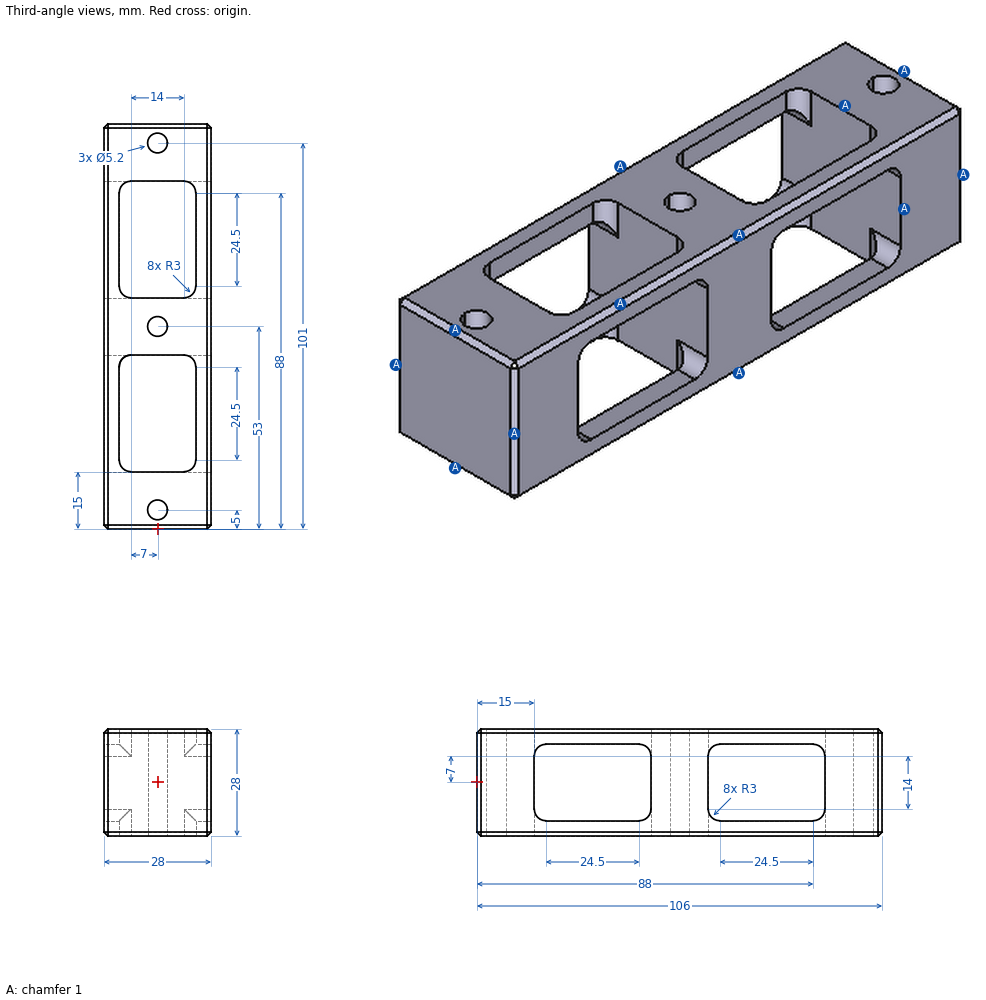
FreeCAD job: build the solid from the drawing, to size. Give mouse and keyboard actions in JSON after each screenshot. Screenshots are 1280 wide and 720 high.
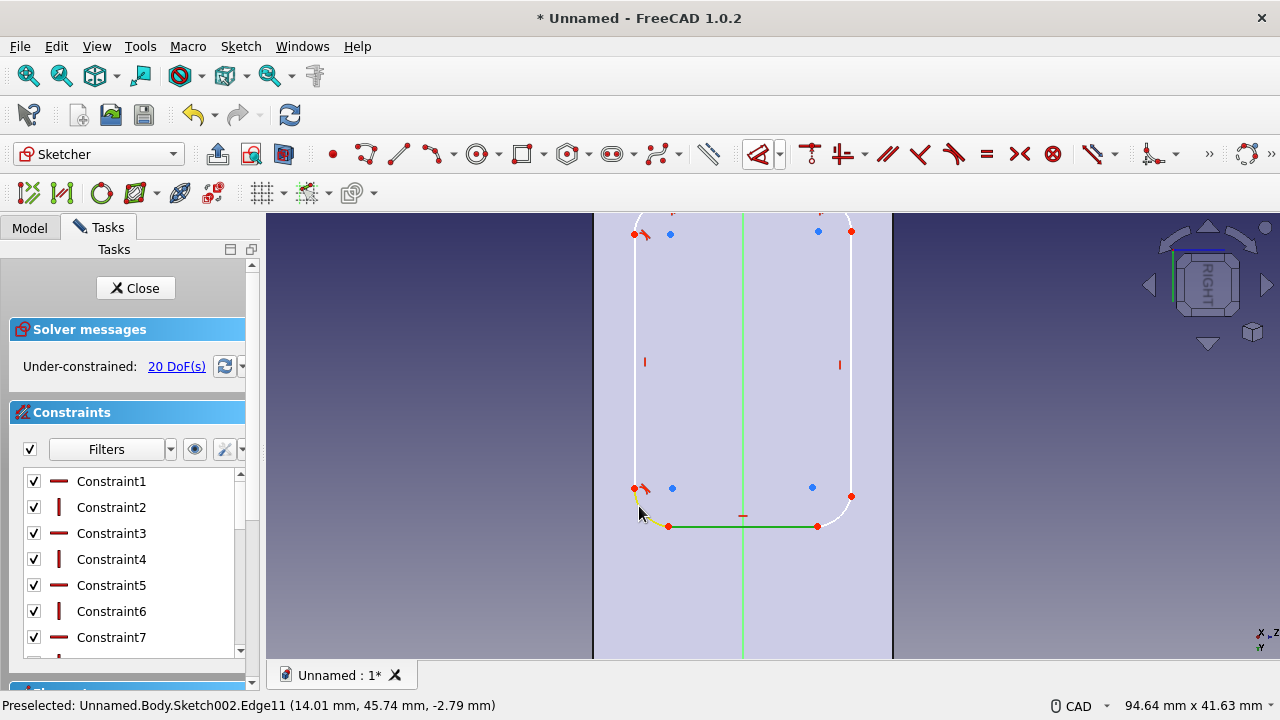
{"action": "left_click", "coordinate": [638, 505]}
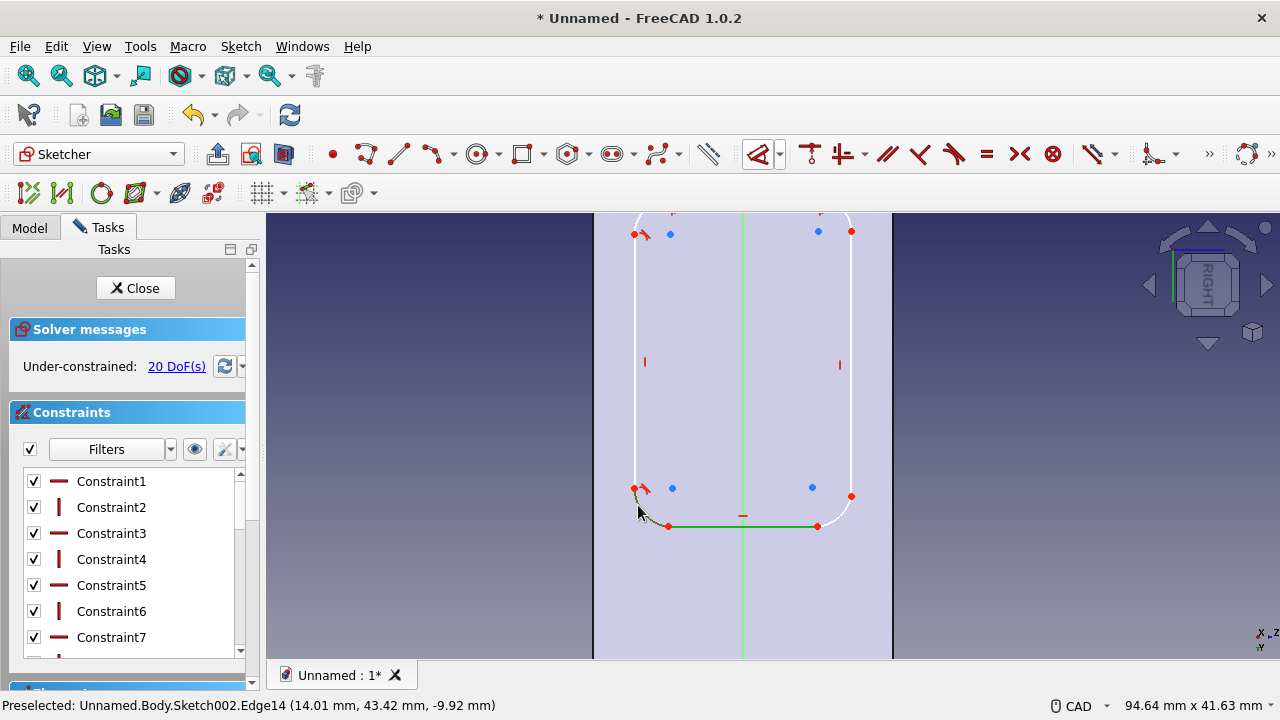
{"action": "left_click", "coordinate": [954, 154]}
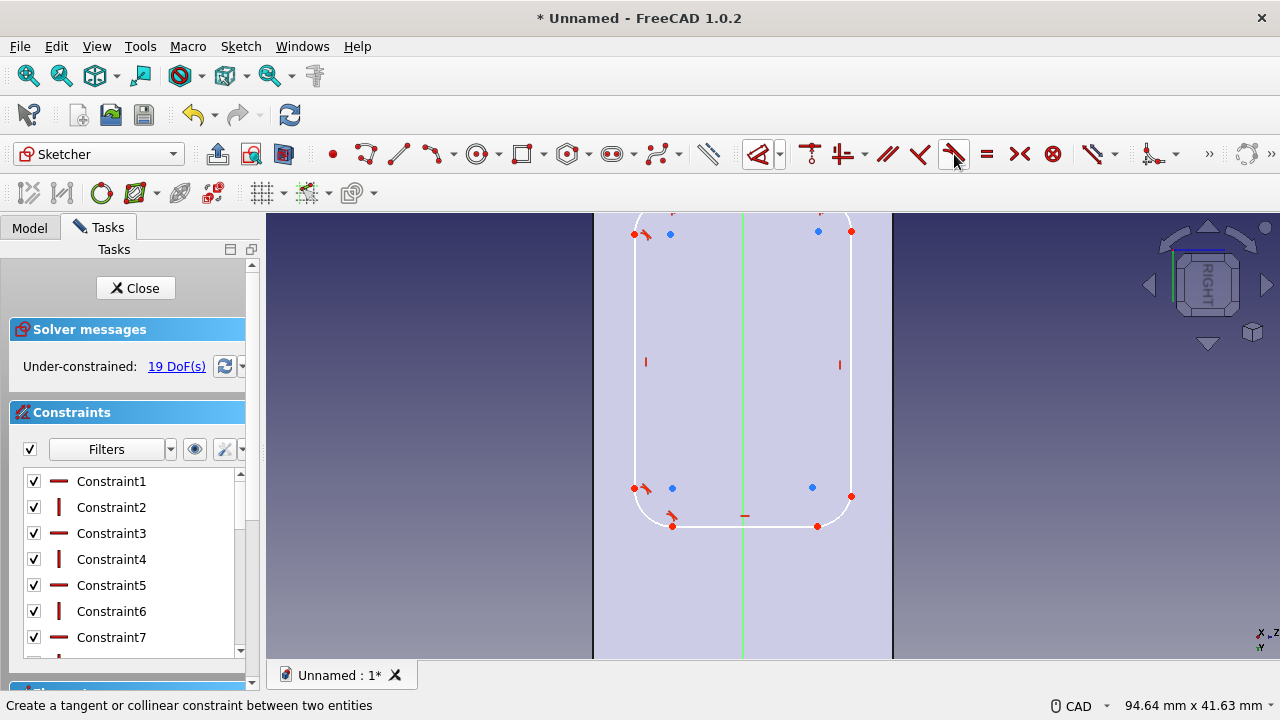
{"action": "left_click", "coordinate": [716, 527]}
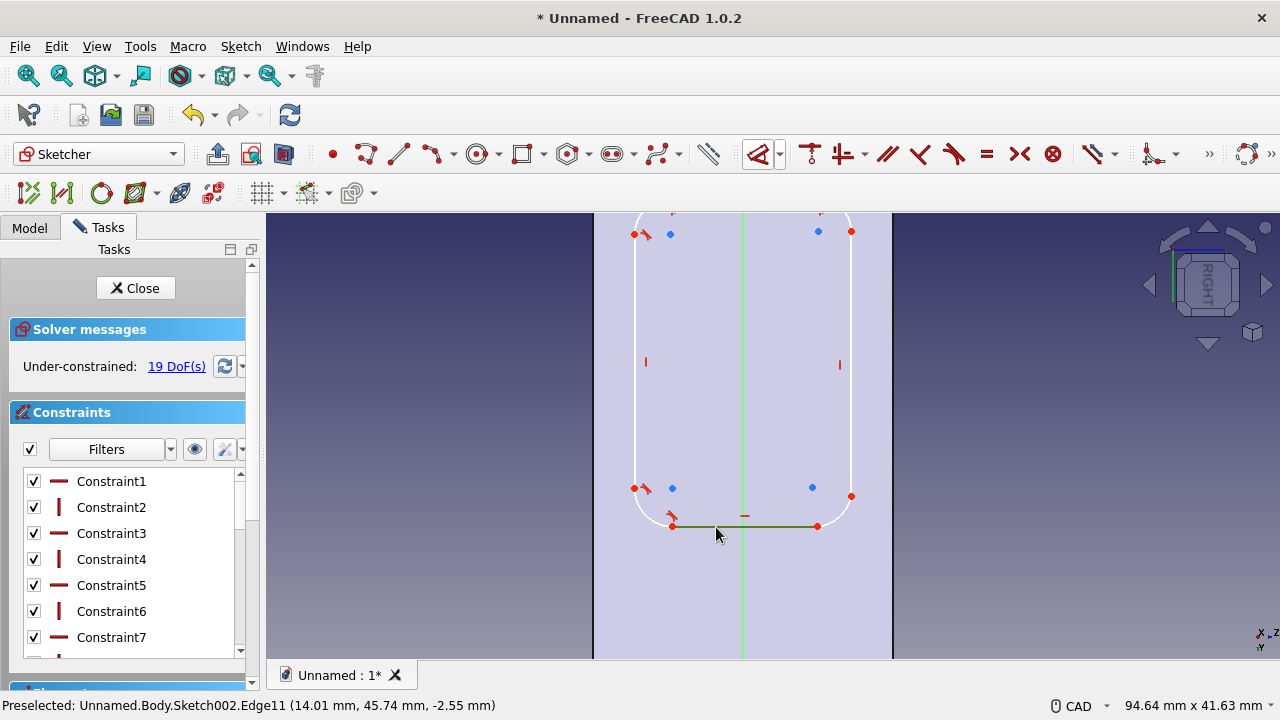
{"action": "left_click", "coordinate": [831, 522]}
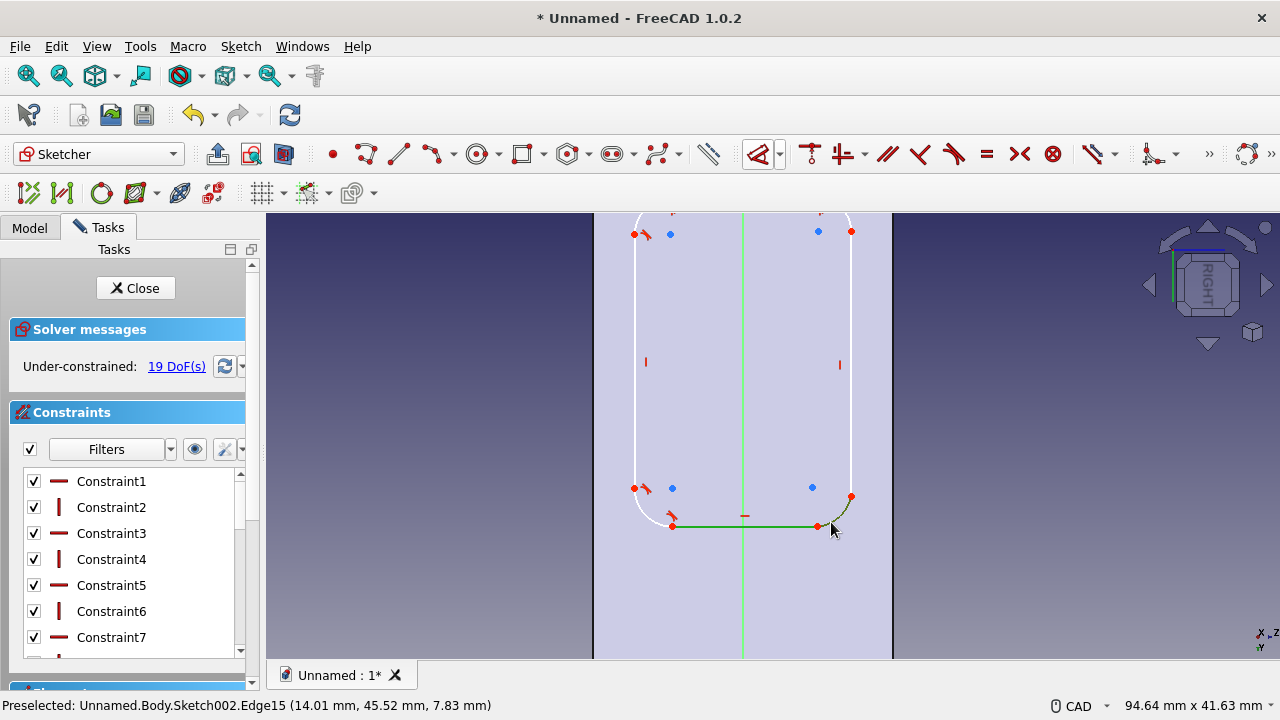
{"action": "left_click", "coordinate": [954, 154]}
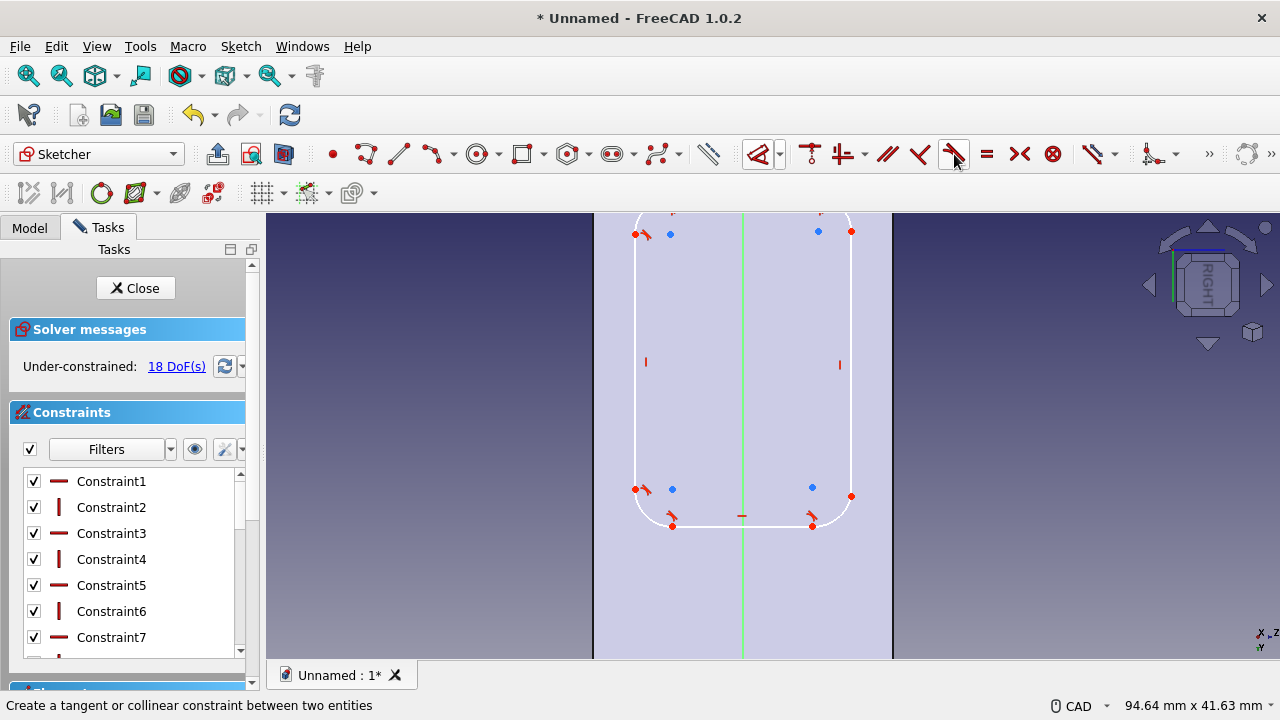
{"action": "left_click", "coordinate": [851, 417]}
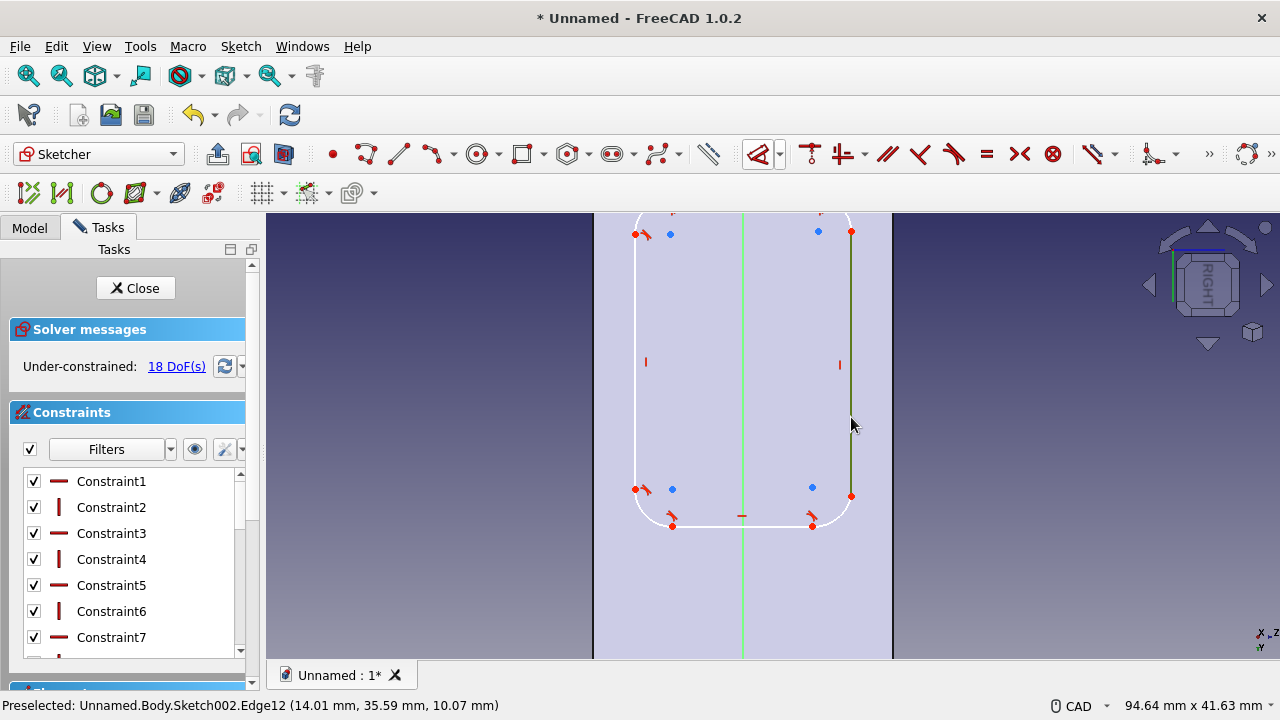
{"action": "left_click", "coordinate": [828, 524]}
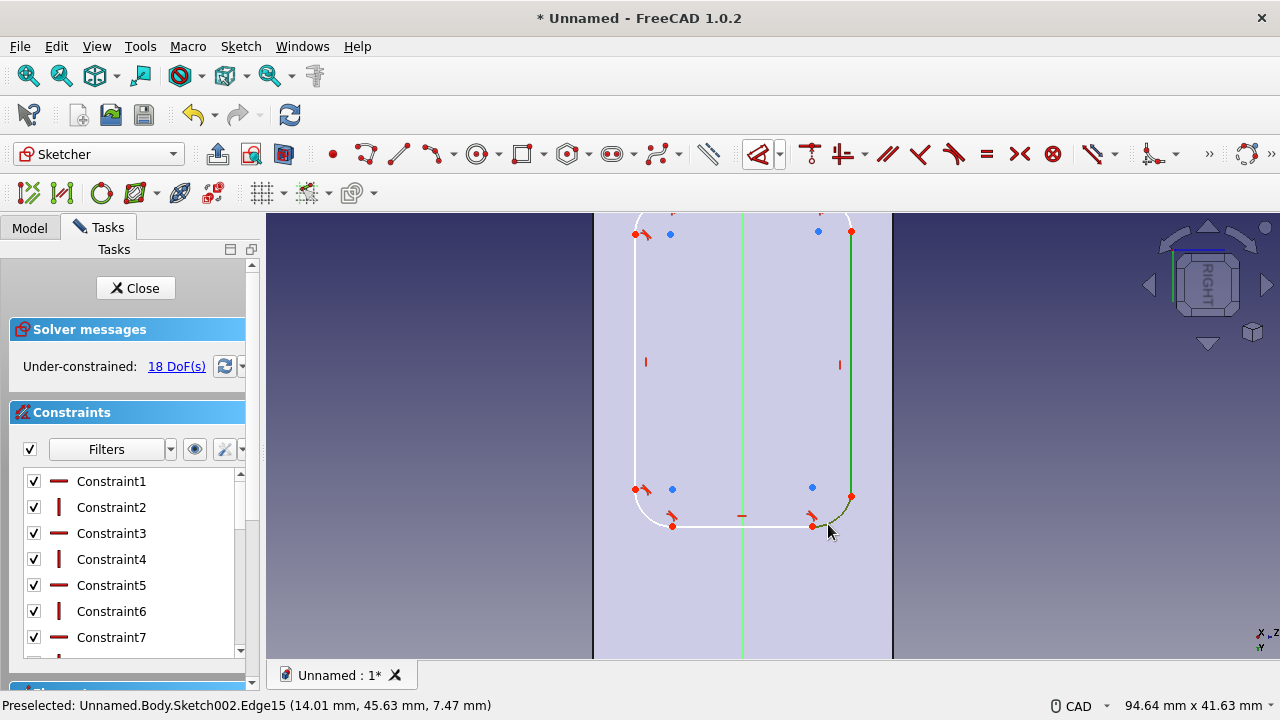
{"action": "left_click", "coordinate": [954, 154]}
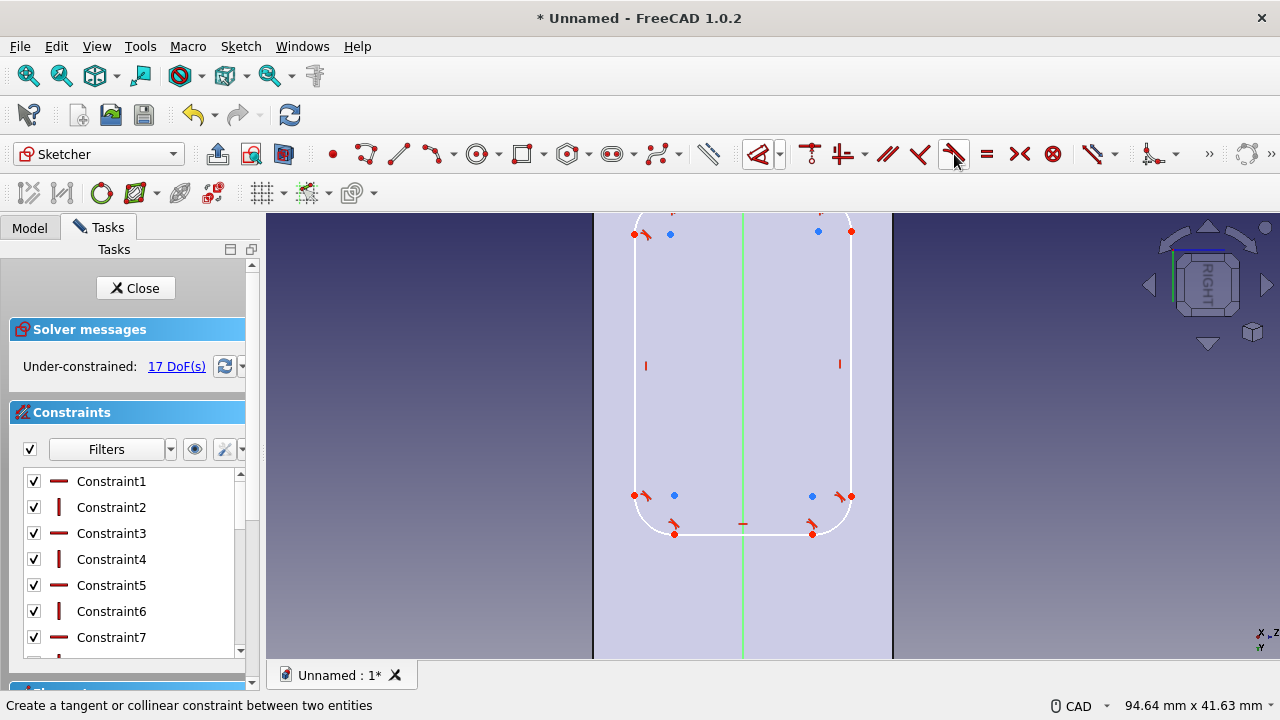
{"action": "left_click", "coordinate": [851, 417]}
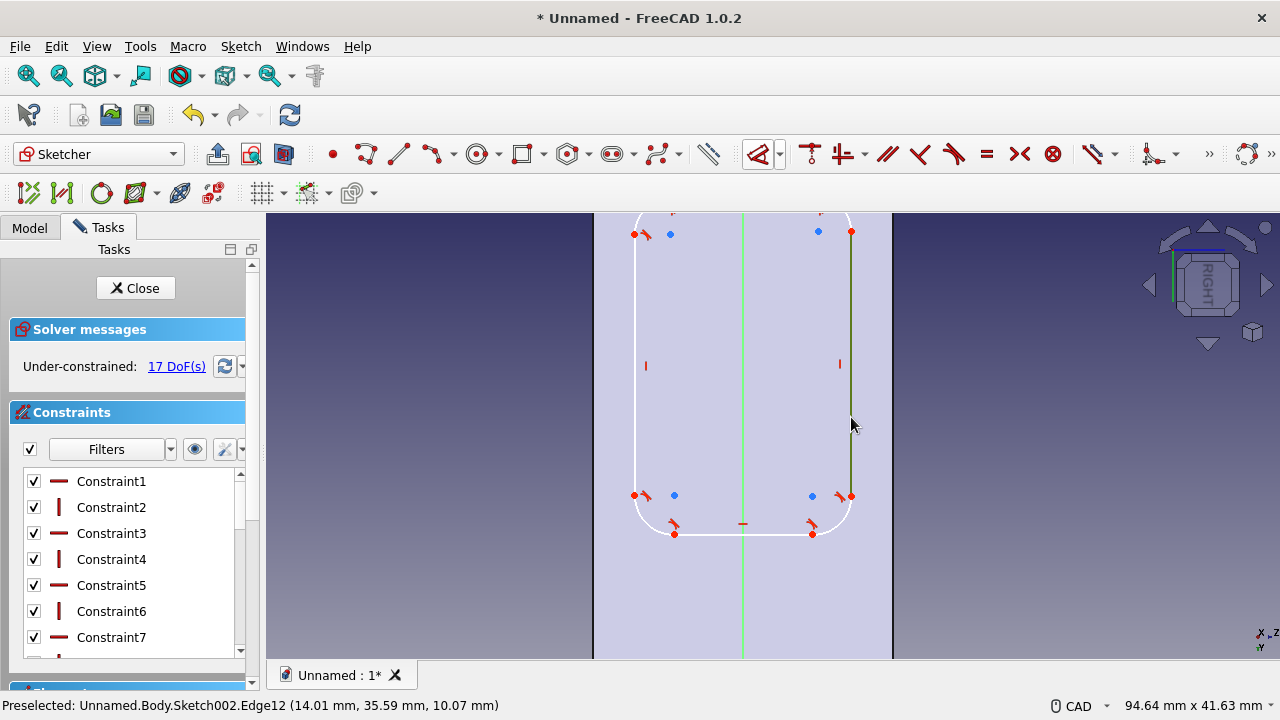
{"action": "scroll", "coordinate": [688, 398], "scroll_direction": "down", "scroll_amount": 6}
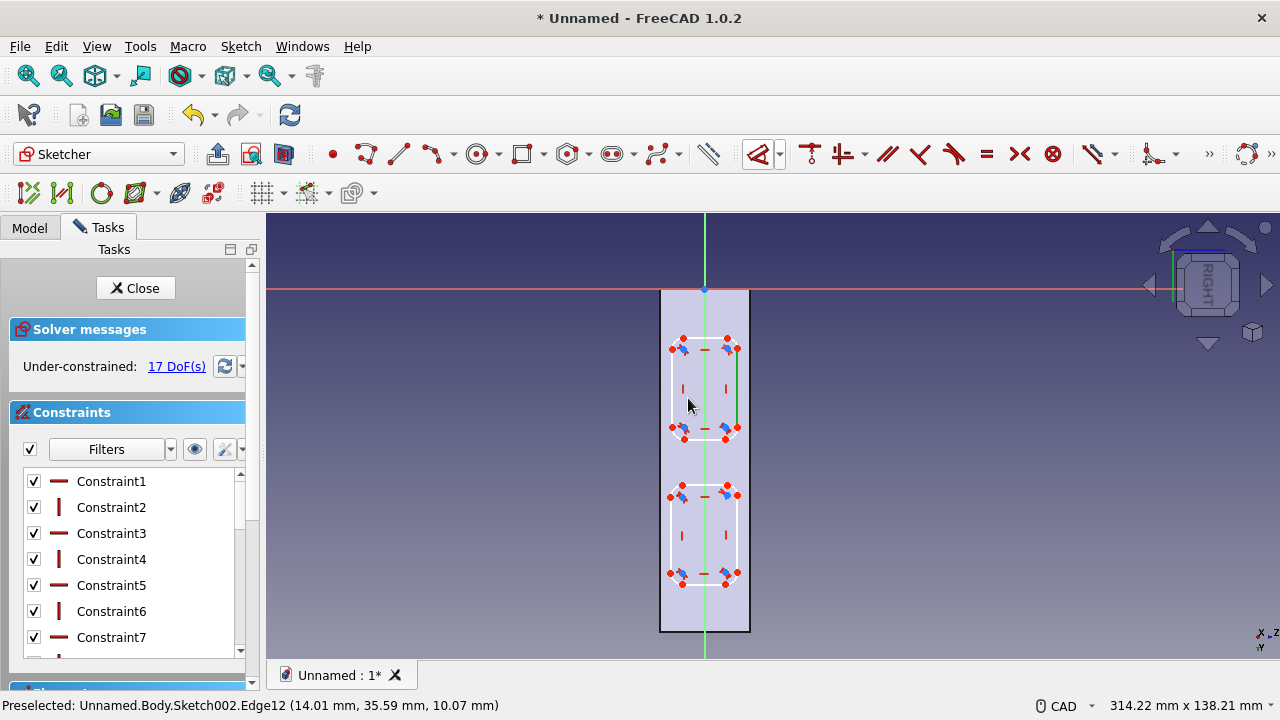
{"action": "scroll", "coordinate": [736, 344], "scroll_direction": "up", "scroll_amount": 6}